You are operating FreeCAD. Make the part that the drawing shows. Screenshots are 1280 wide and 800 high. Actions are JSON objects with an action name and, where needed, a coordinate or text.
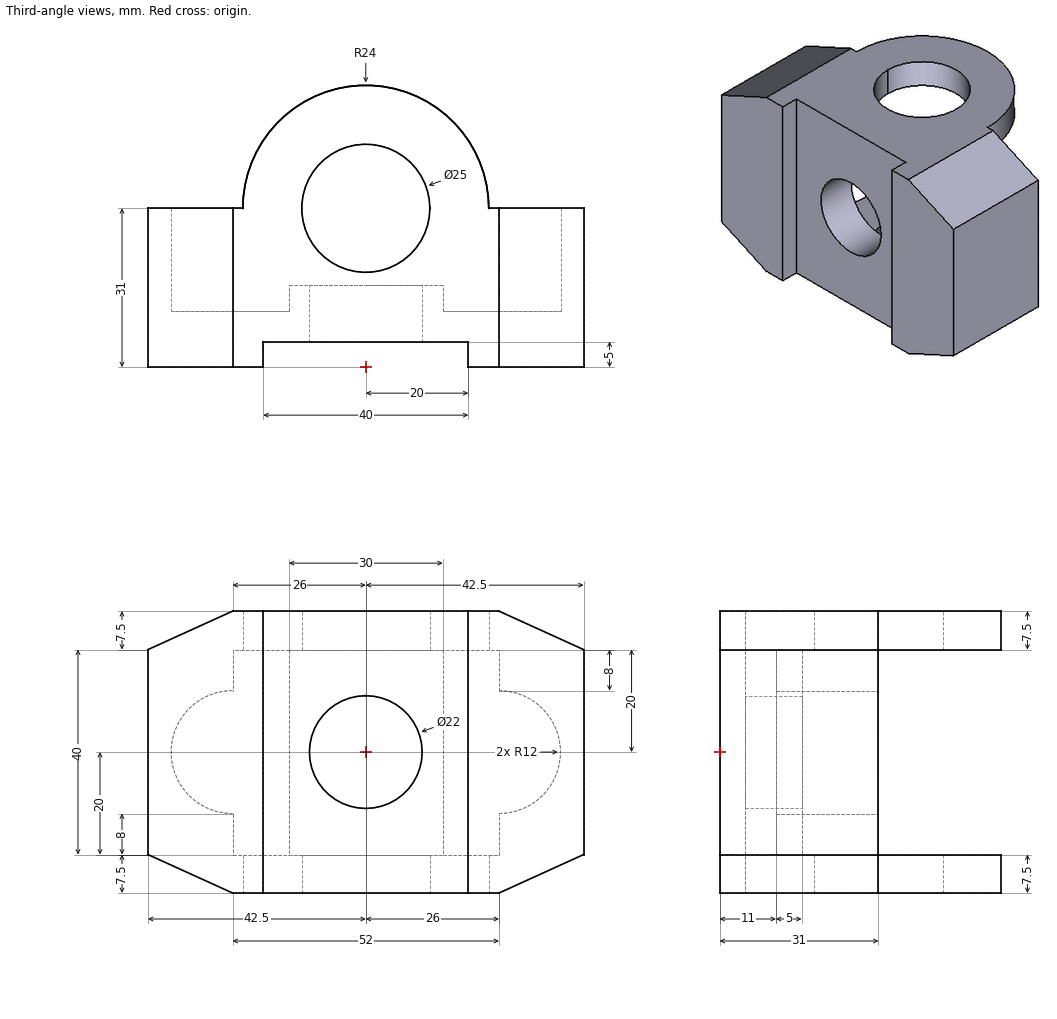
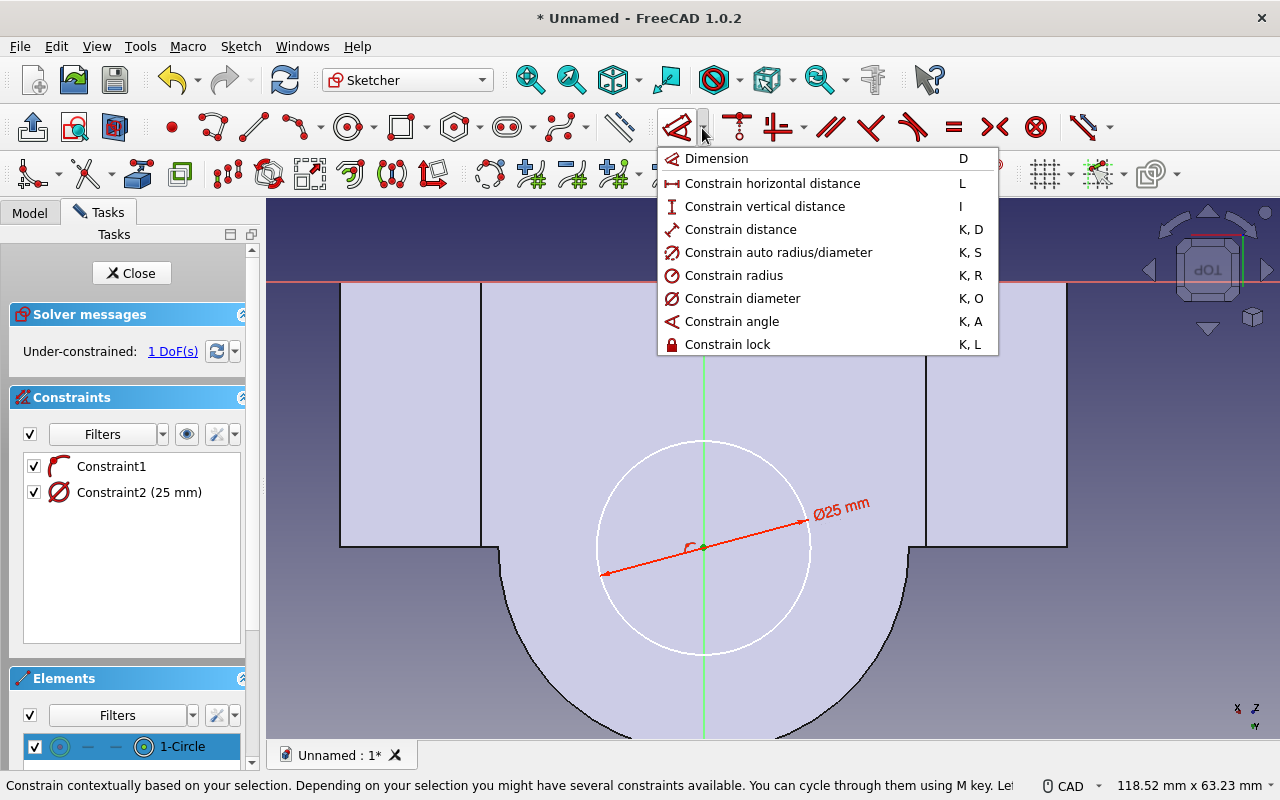
{"action": "left_click", "coordinate": [828, 206]}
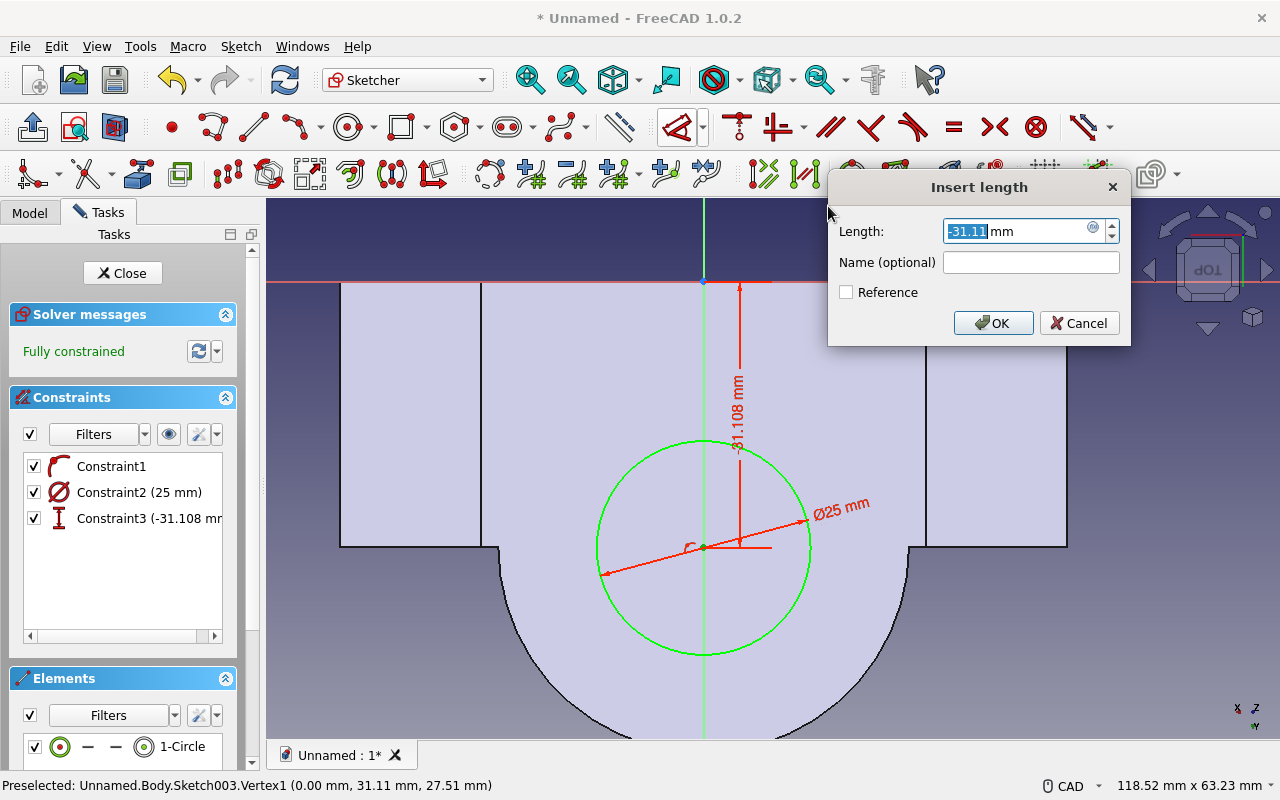
{"action": "type", "text": "-31"}
{"action": "key", "text": "Return"}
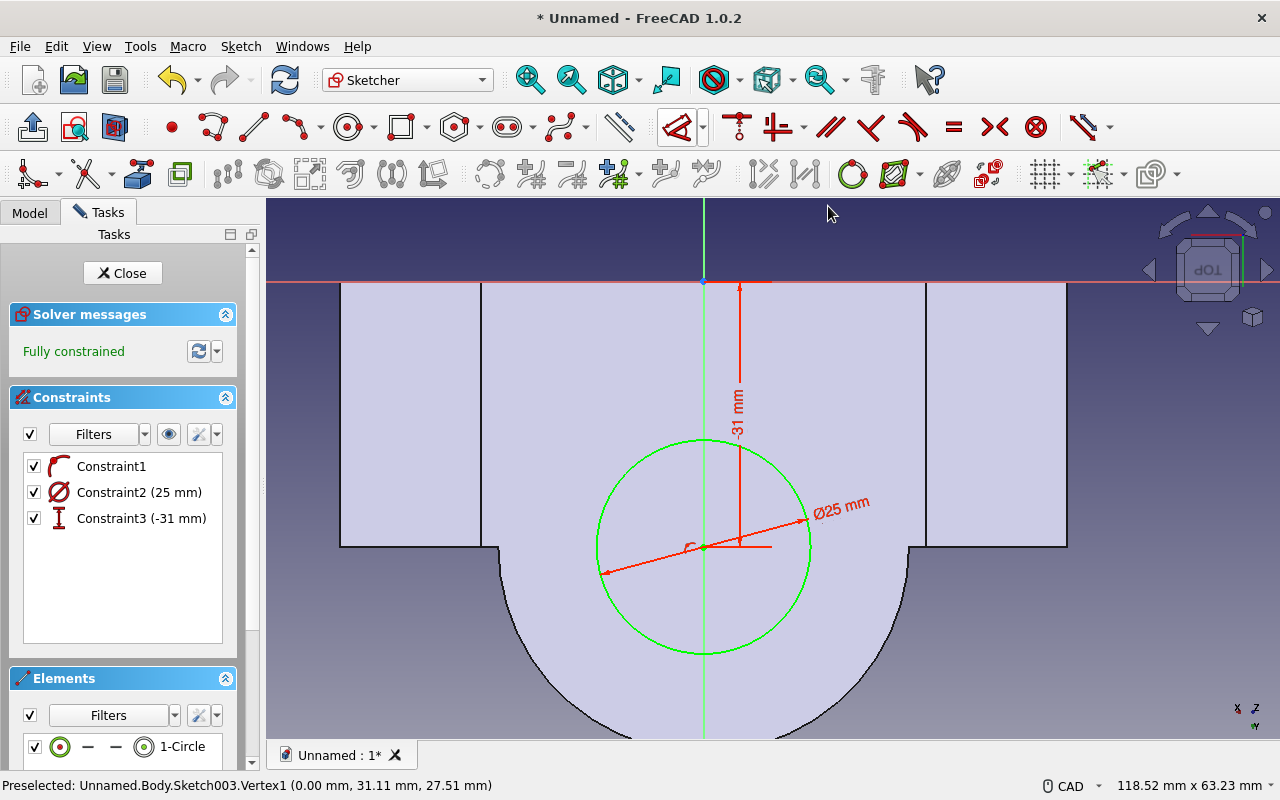
{"action": "left_click", "coordinate": [123, 273]}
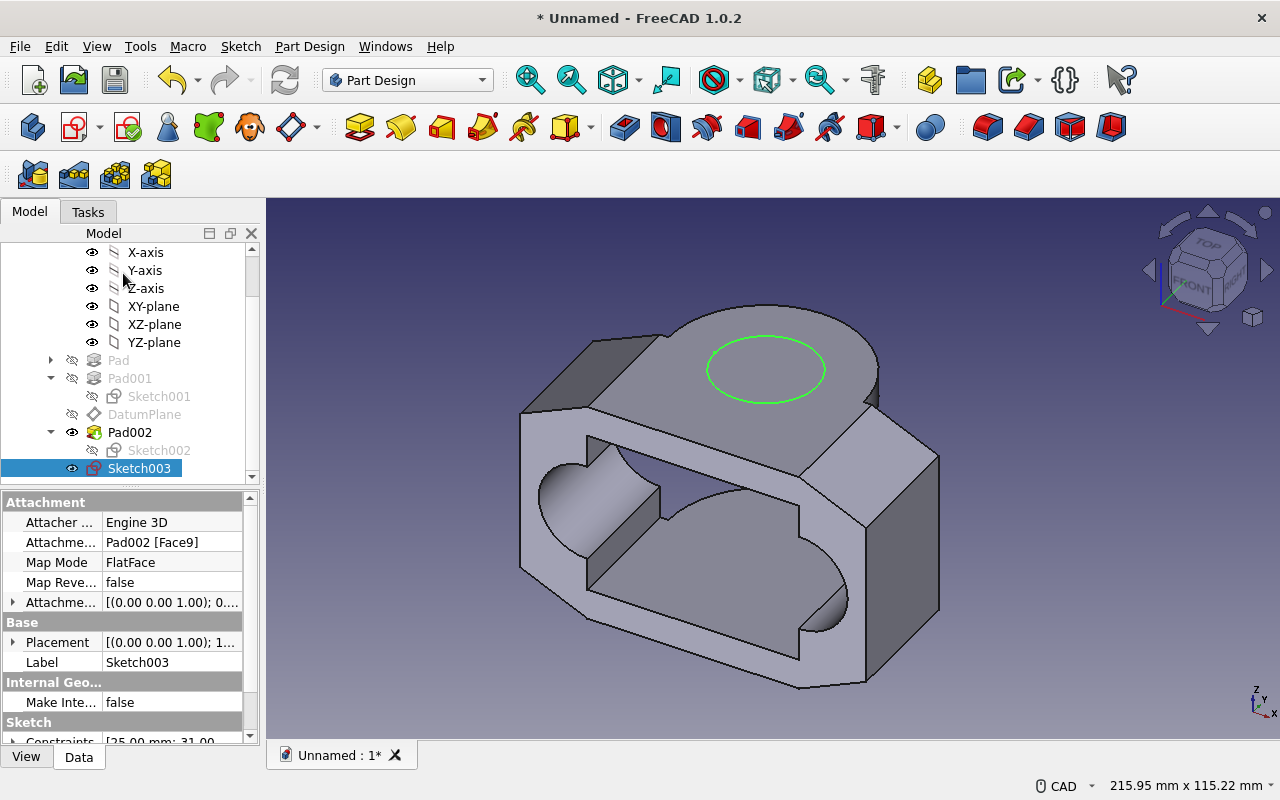
{"action": "left_click", "coordinate": [625, 128]}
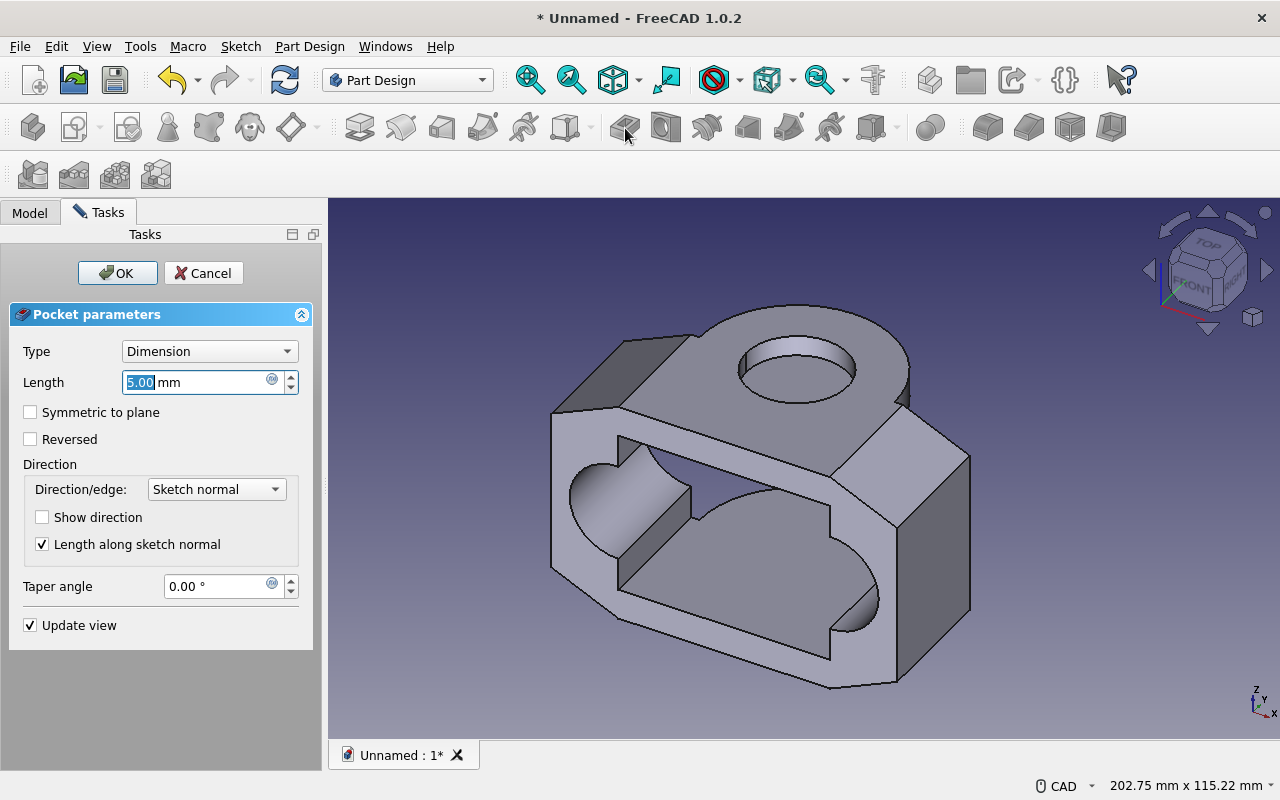
{"action": "left_click", "coordinate": [210, 352]}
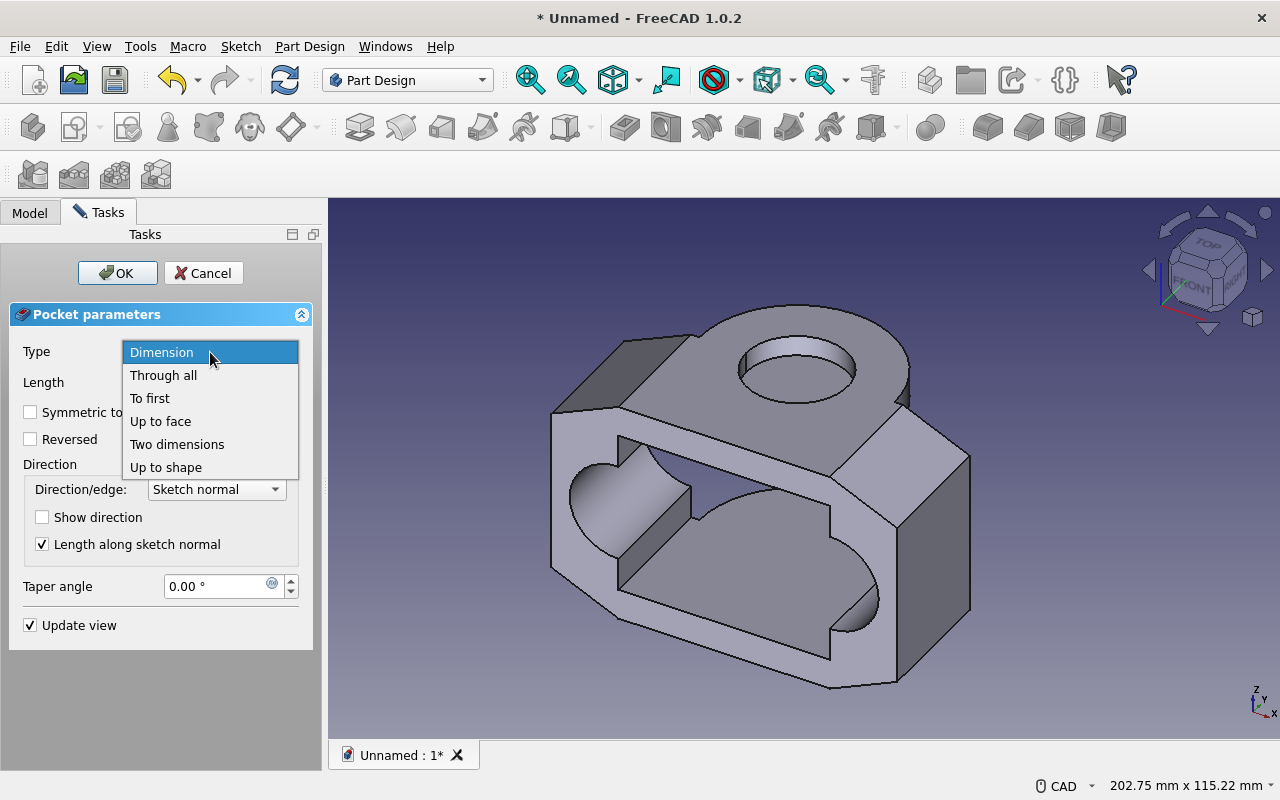
{"action": "left_click", "coordinate": [208, 376]}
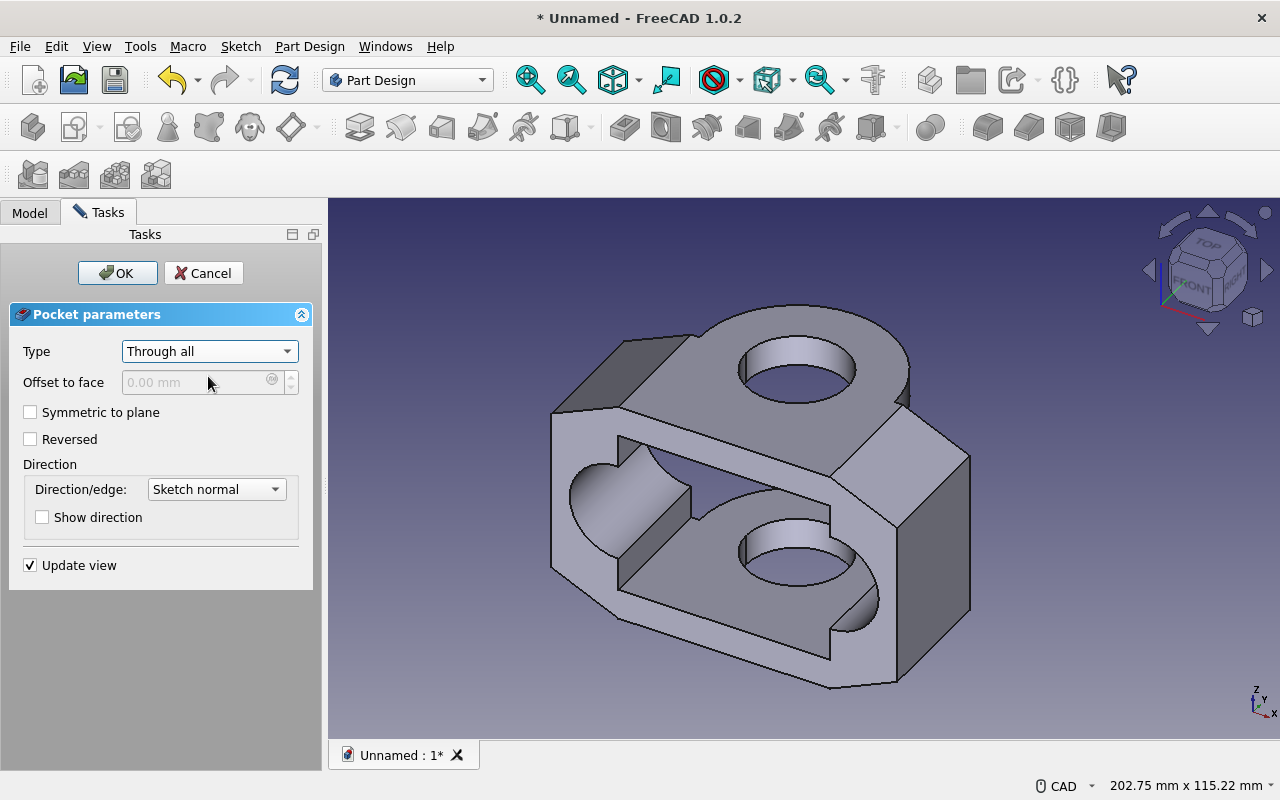
{"action": "left_click", "coordinate": [118, 273]}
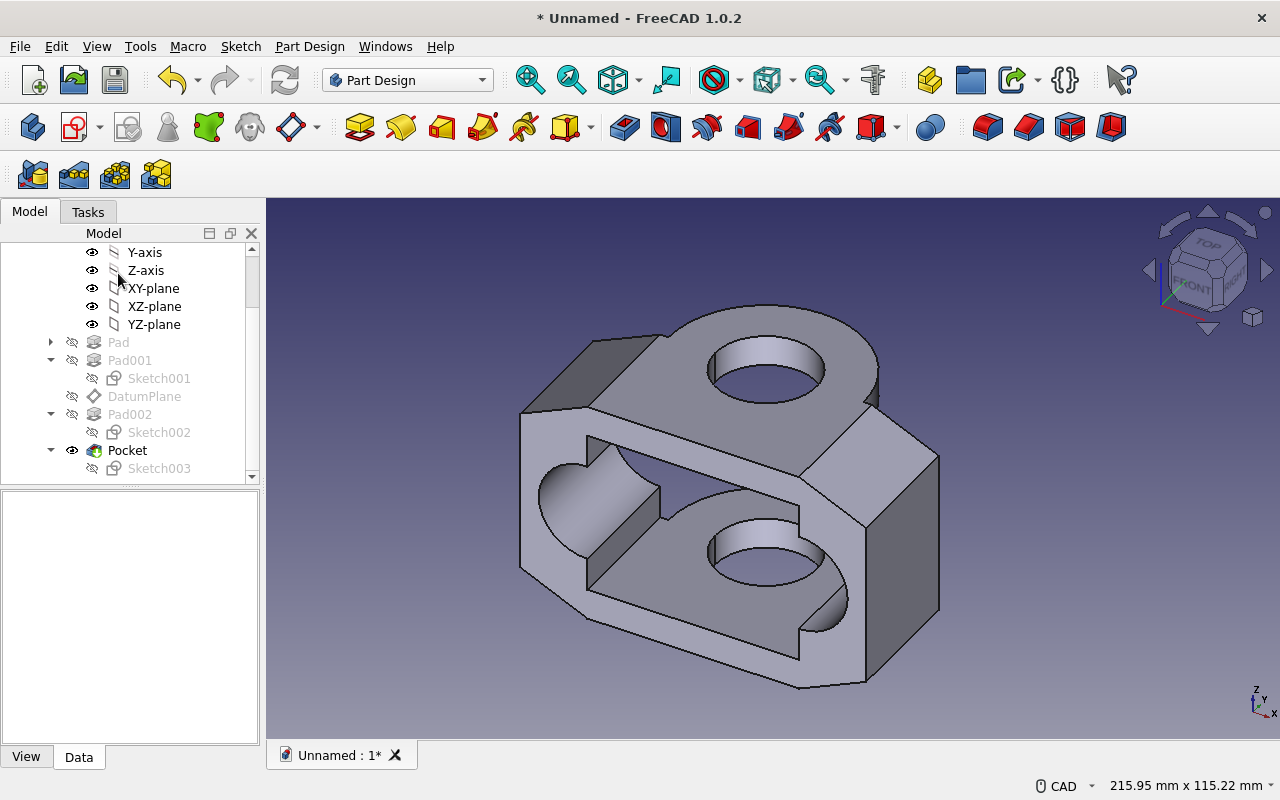
{"action": "left_click", "coordinate": [841, 535]}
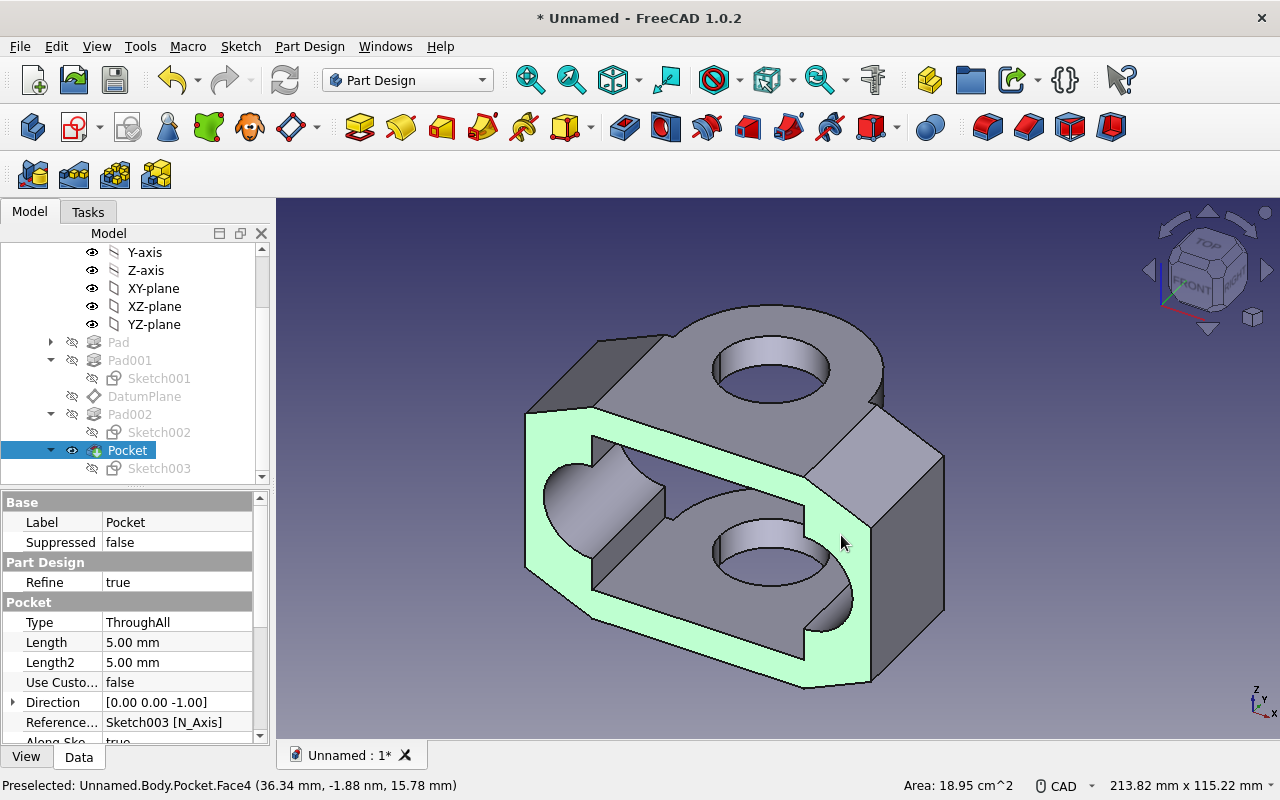
{"action": "left_click", "coordinate": [74, 128]}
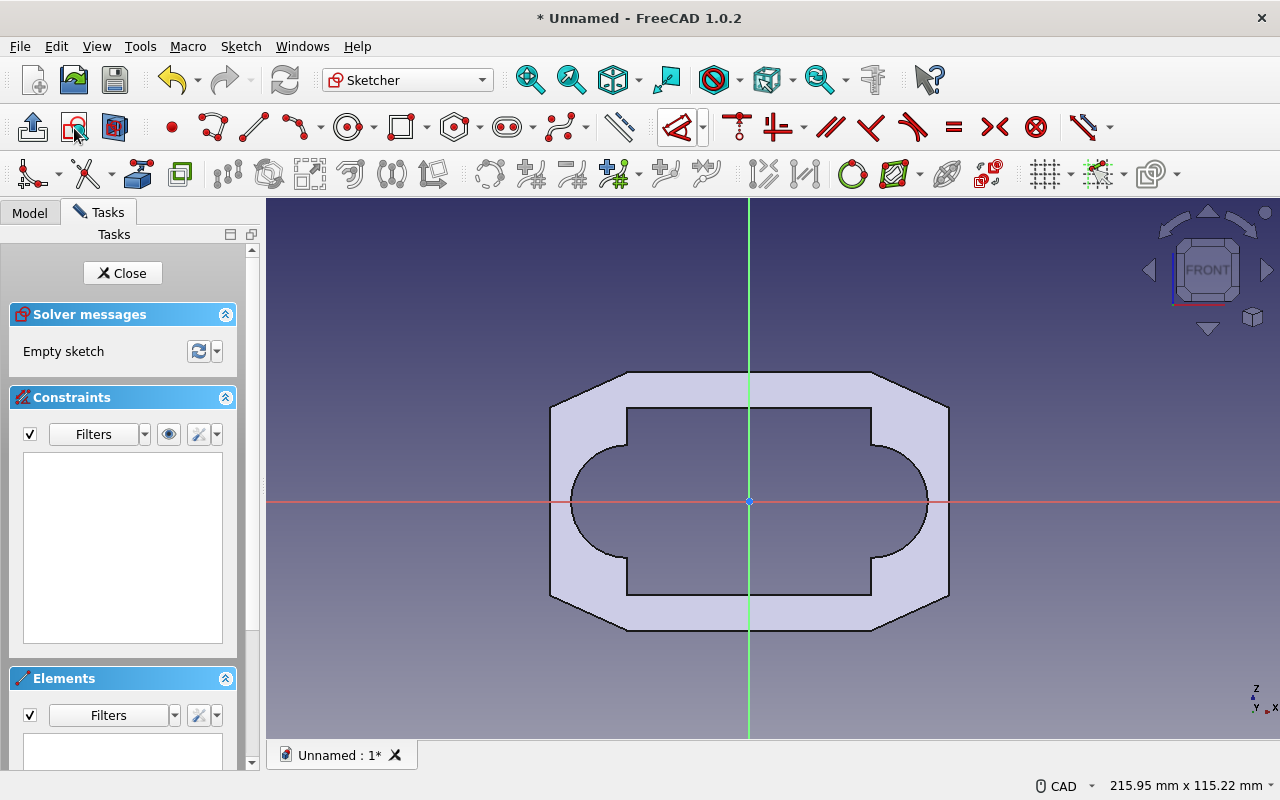
{"action": "key", "text": "g m"}